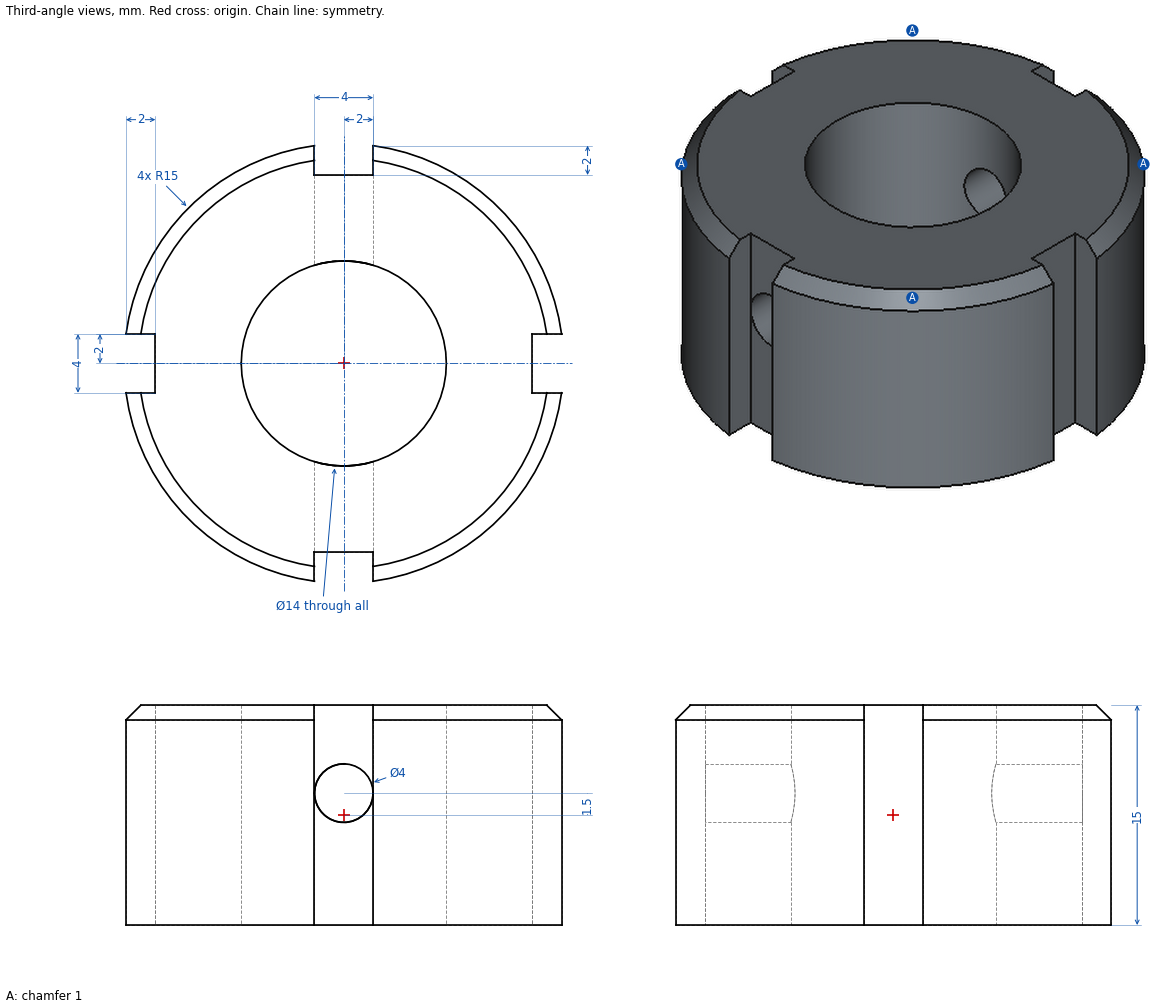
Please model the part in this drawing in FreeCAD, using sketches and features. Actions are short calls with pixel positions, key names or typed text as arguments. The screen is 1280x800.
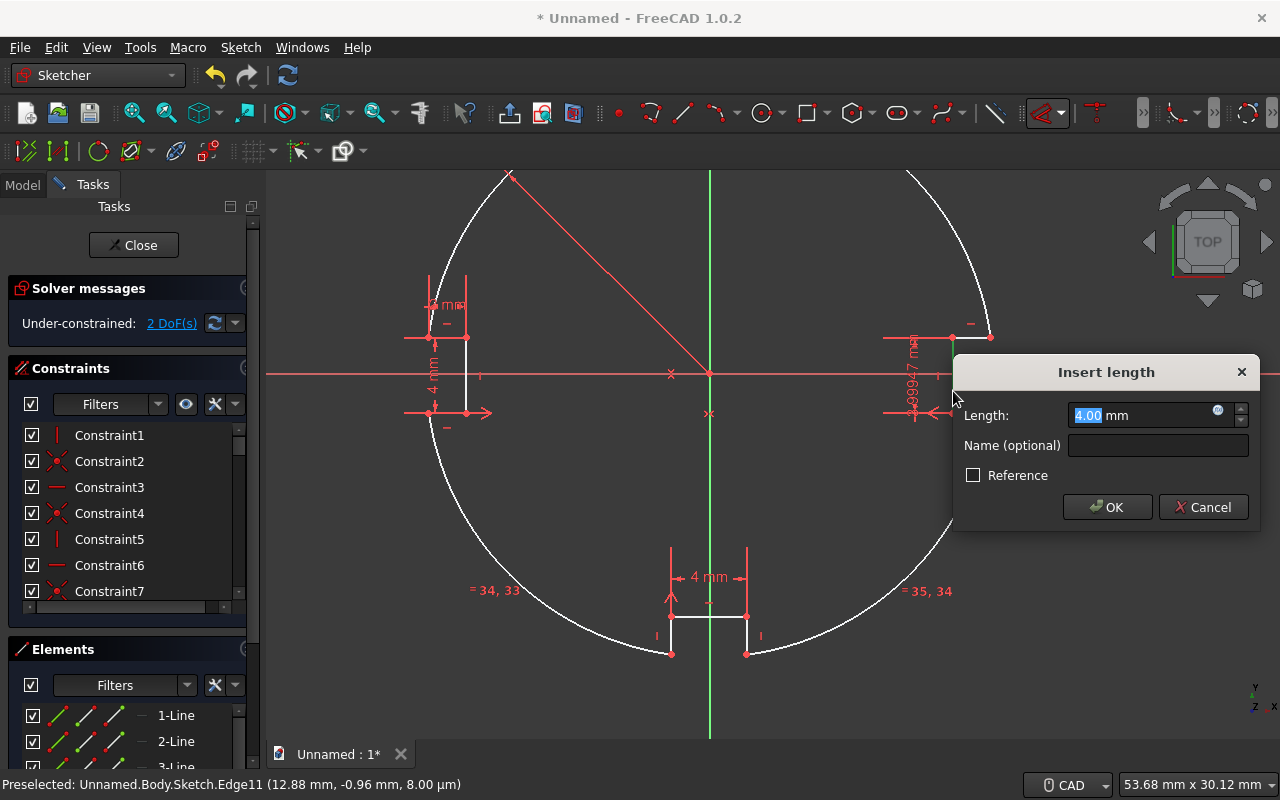
text(4)
key(Return)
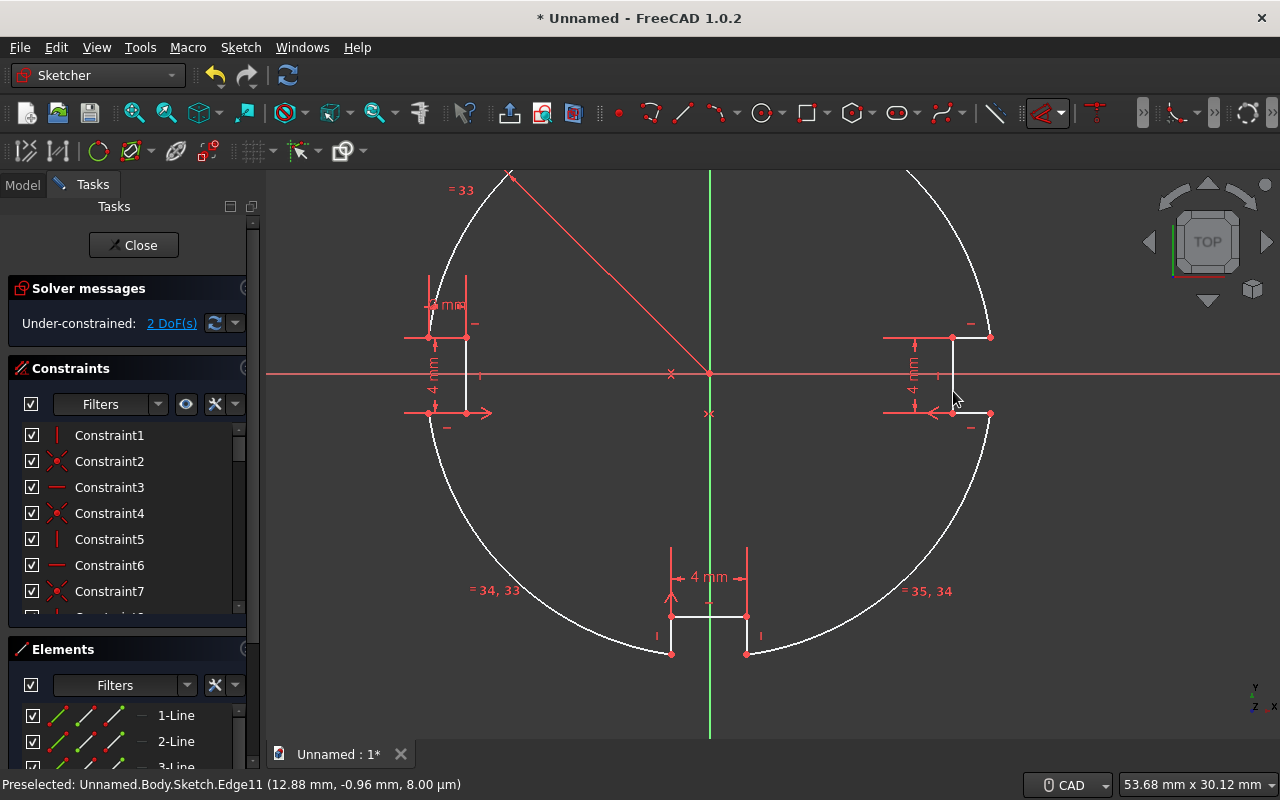
scroll(694, 618, down, 2)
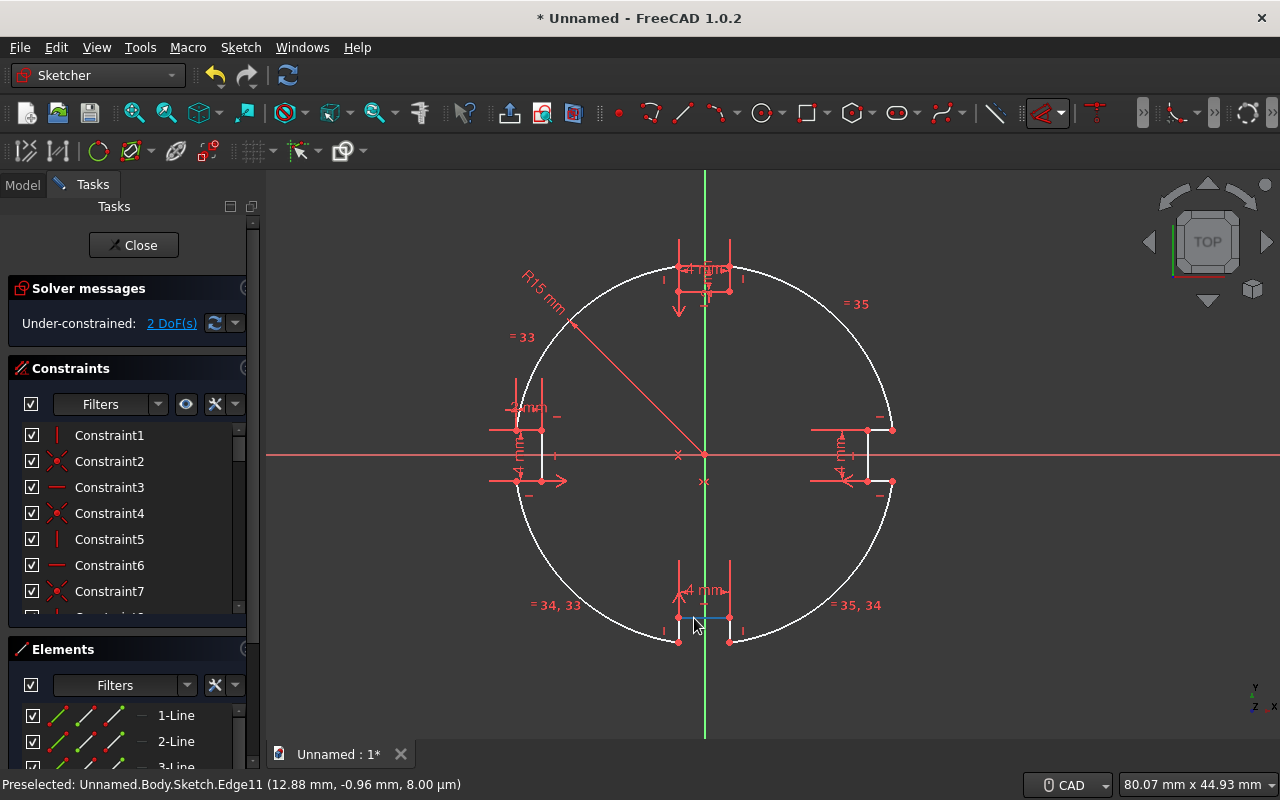
scroll(730, 266, up, 3)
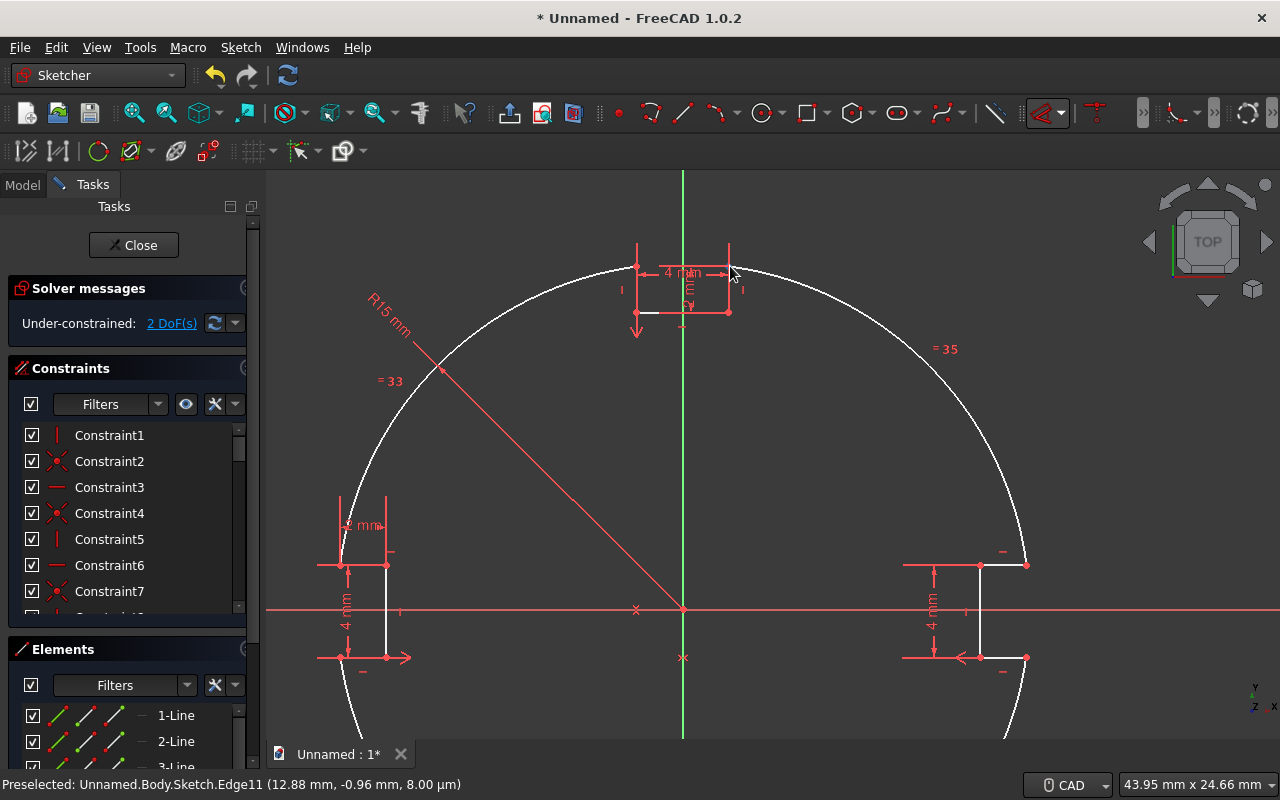
click(729, 266)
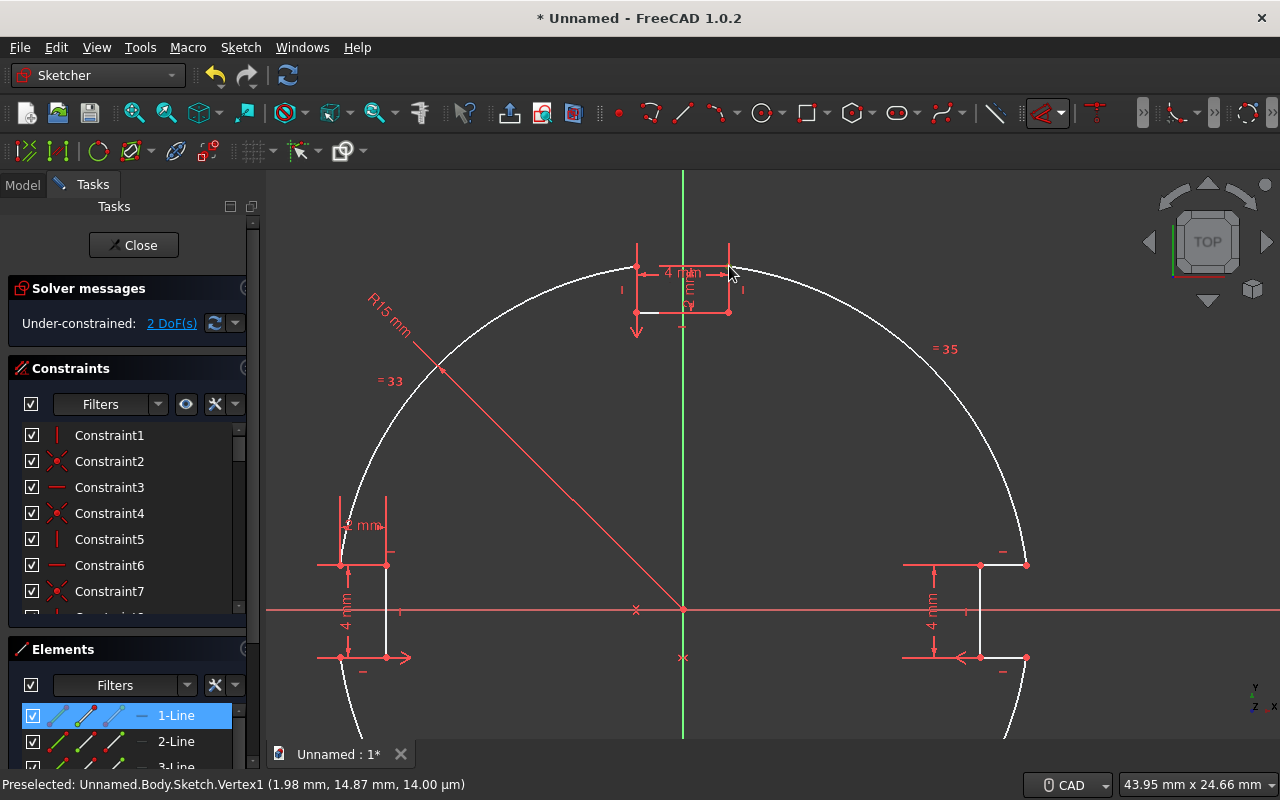
key(l)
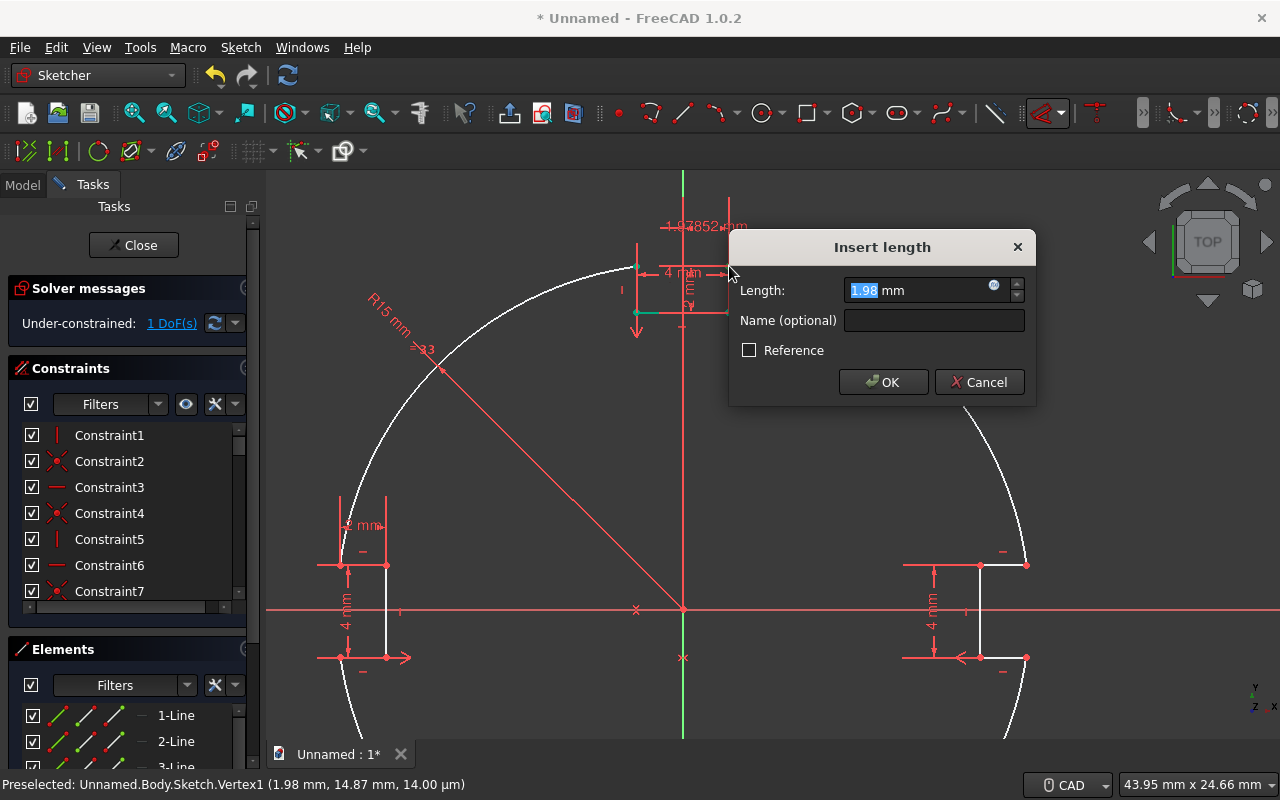
text(2)
key(Return)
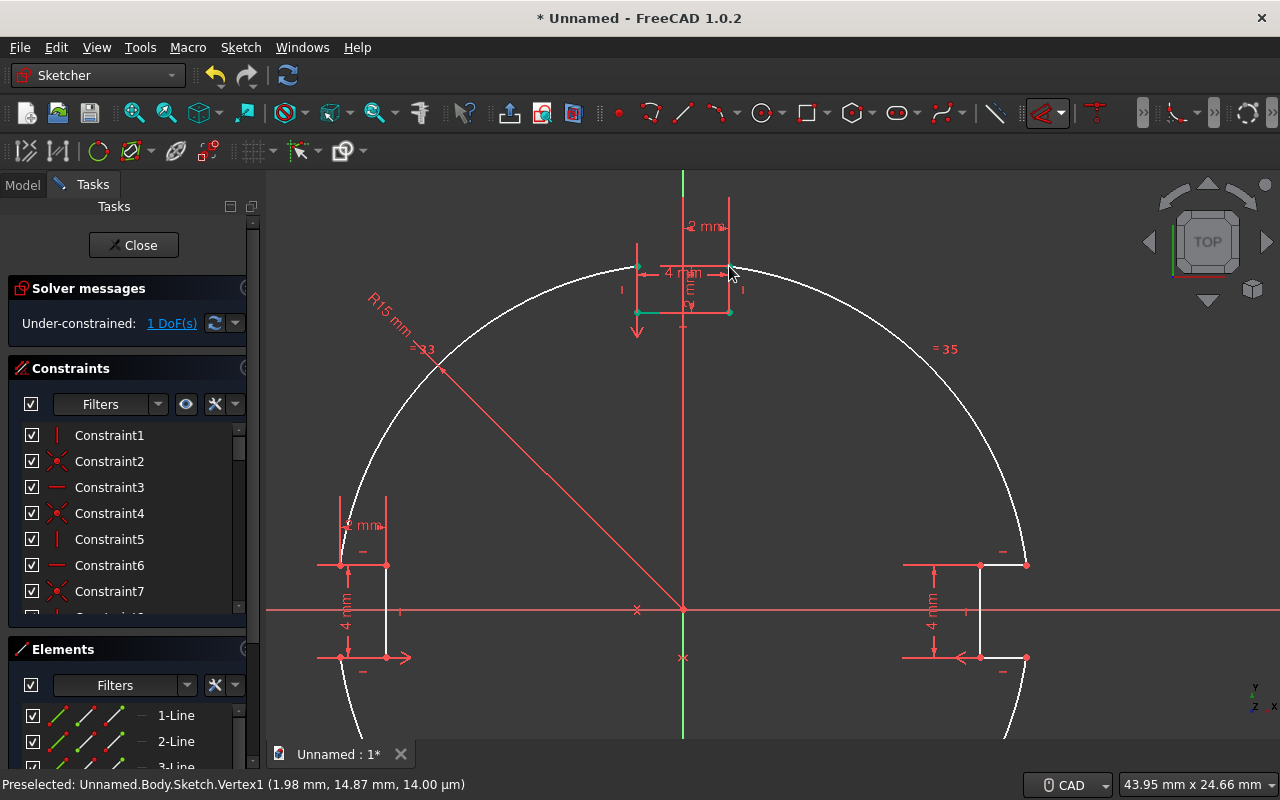
click(340, 565)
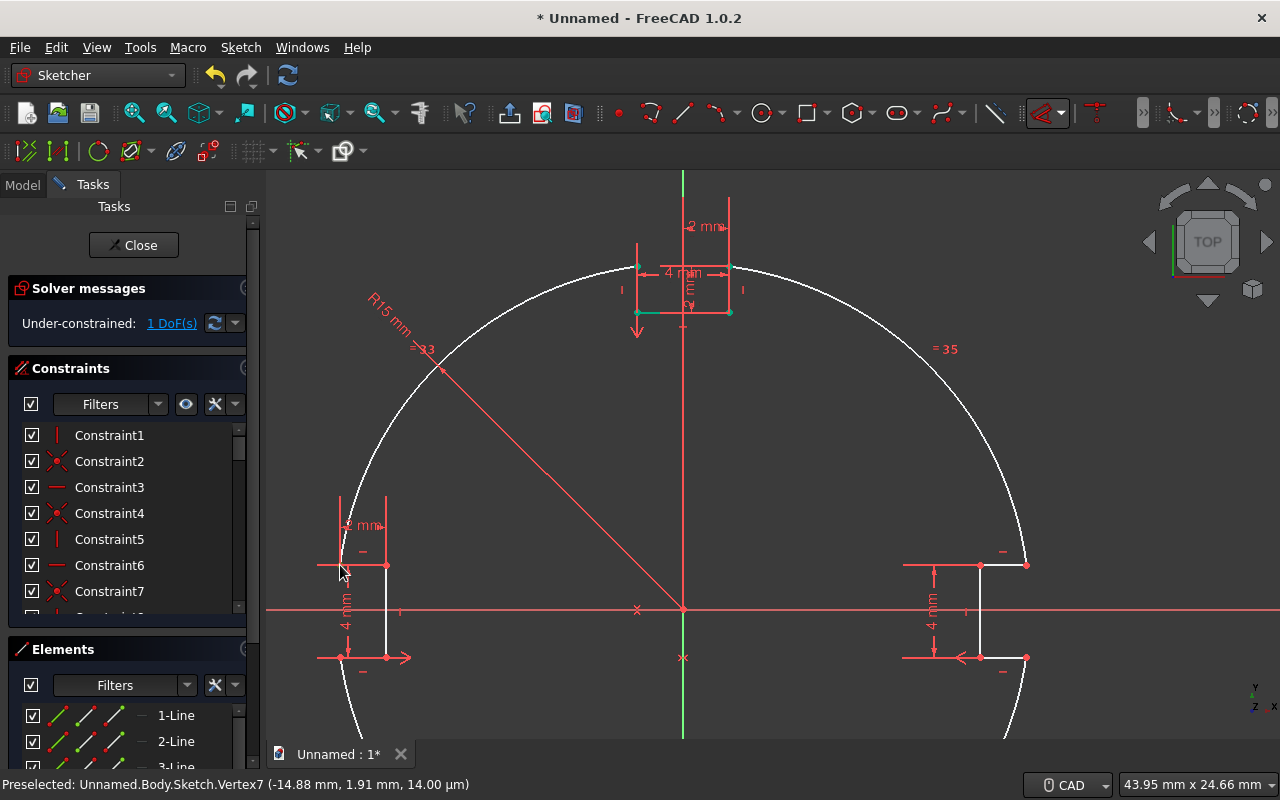
key(i)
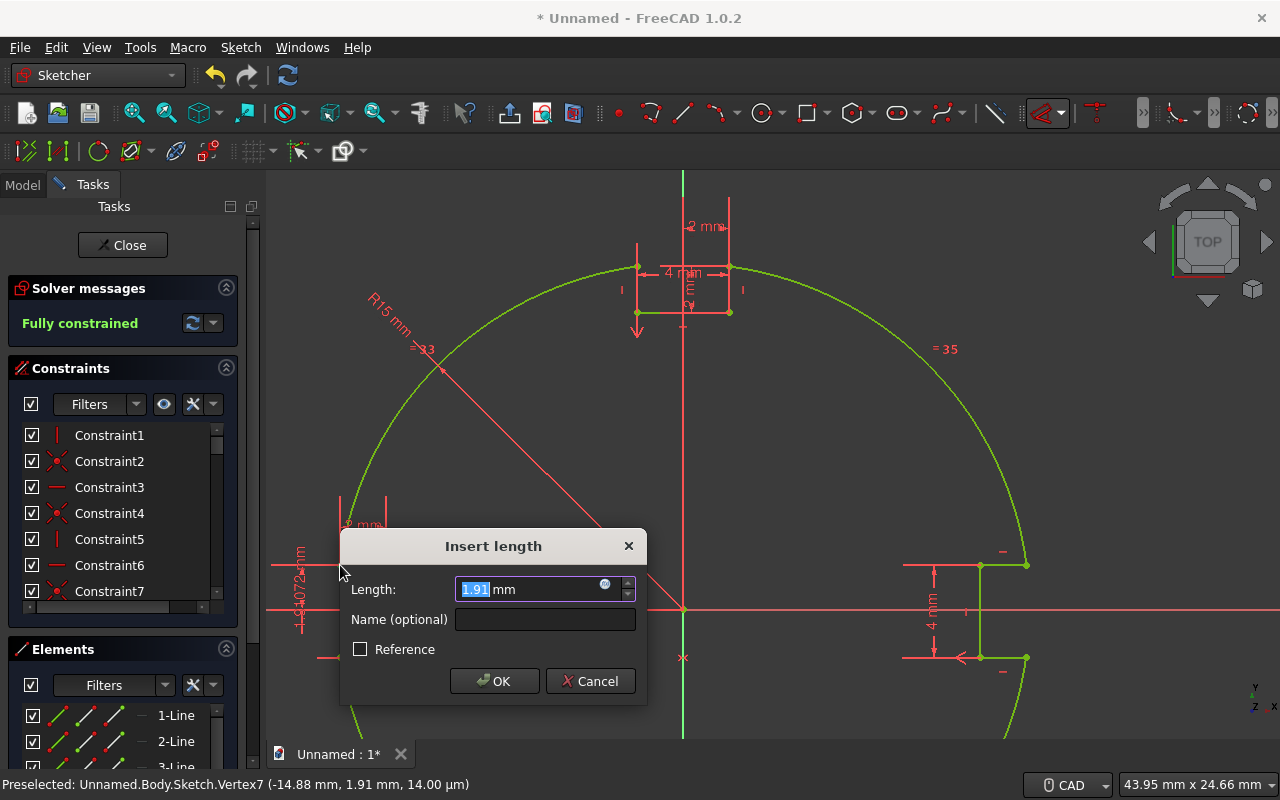
text(2)
key(Return)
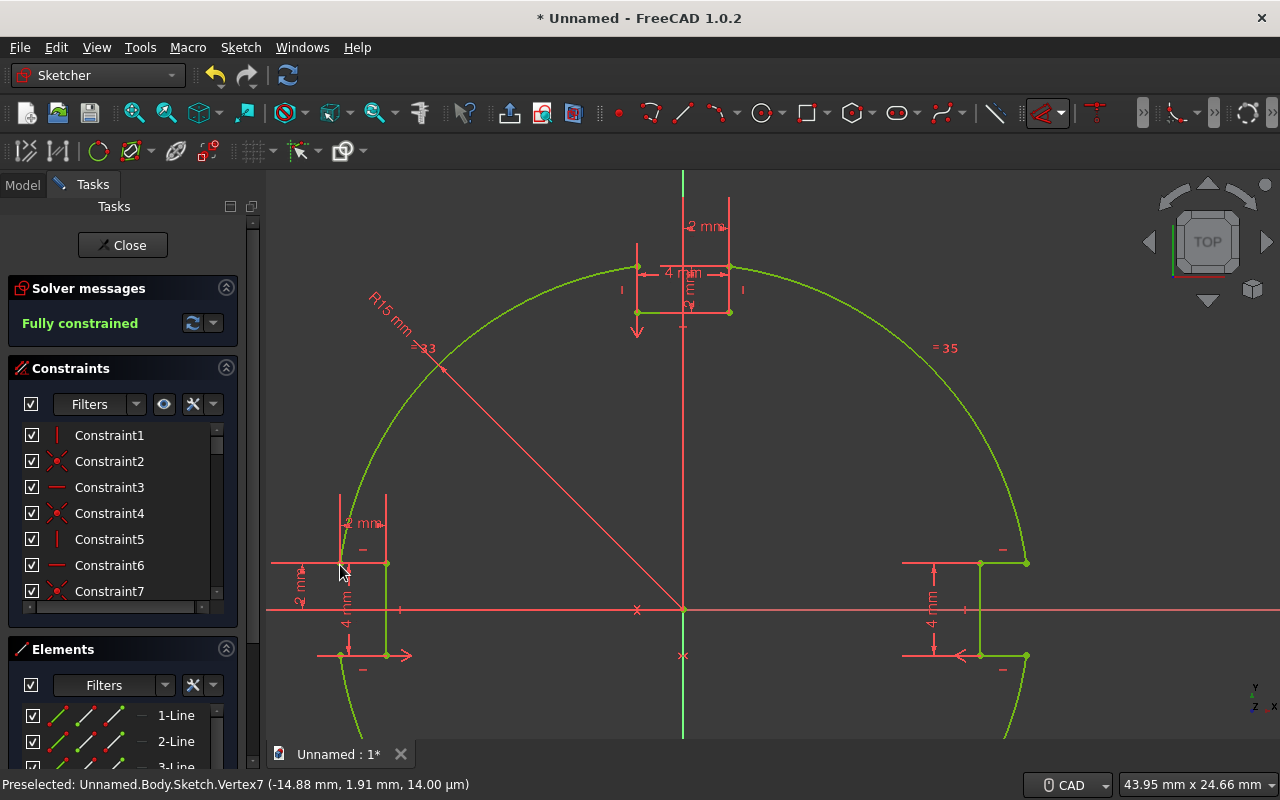
click(123, 245)